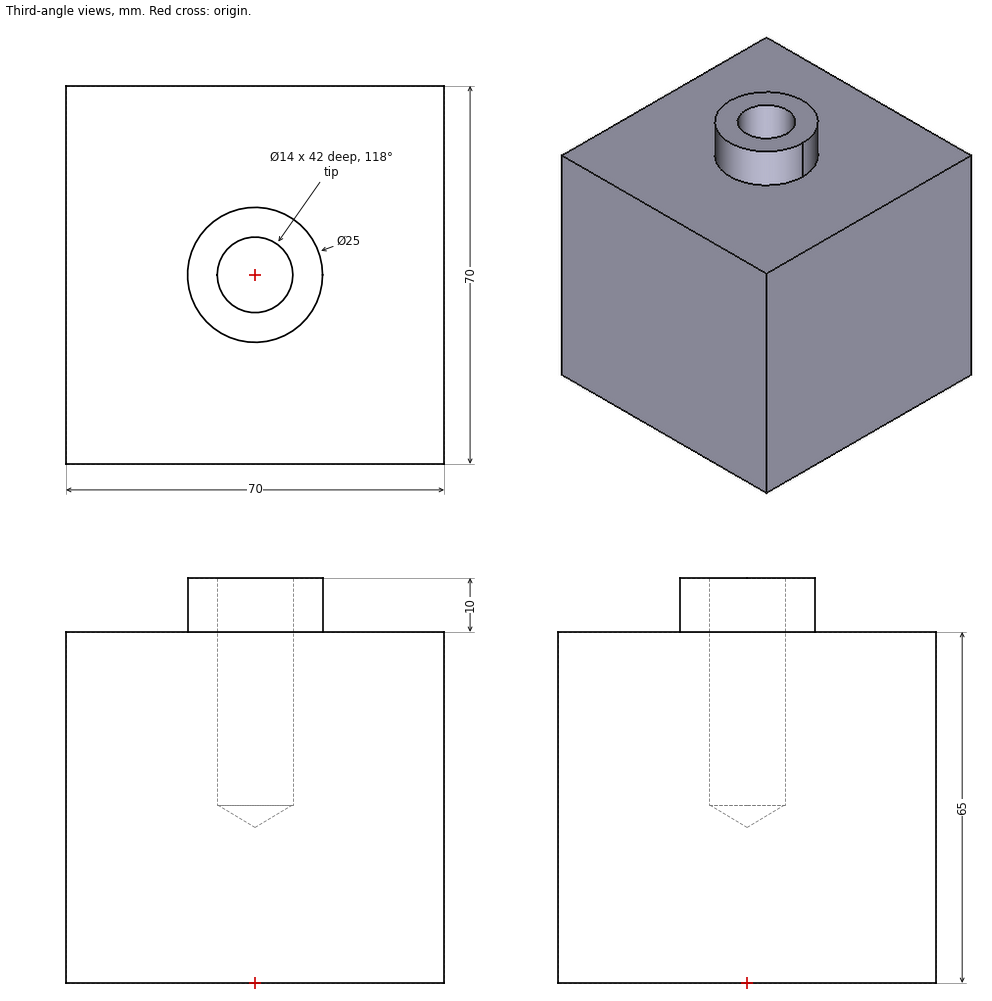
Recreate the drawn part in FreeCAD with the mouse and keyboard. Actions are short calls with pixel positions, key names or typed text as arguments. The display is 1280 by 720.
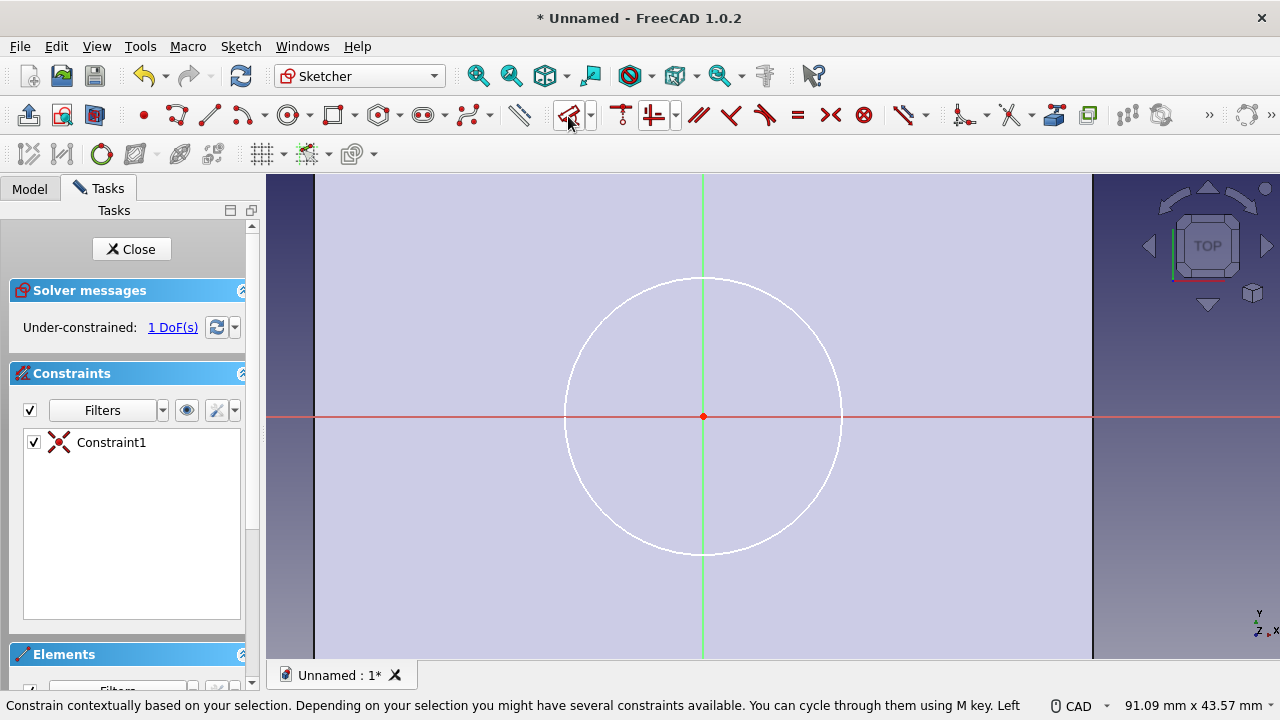
click(801, 318)
click(824, 295)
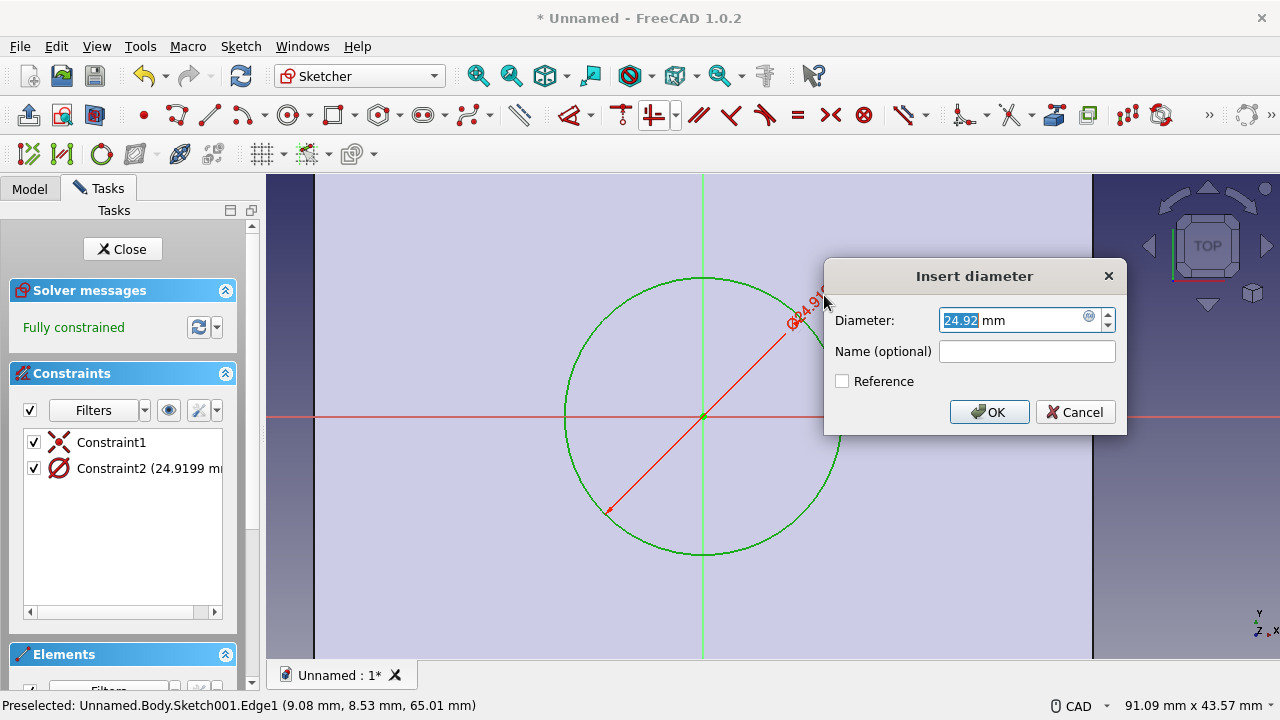
text(25)
key(Return)
key(Escape)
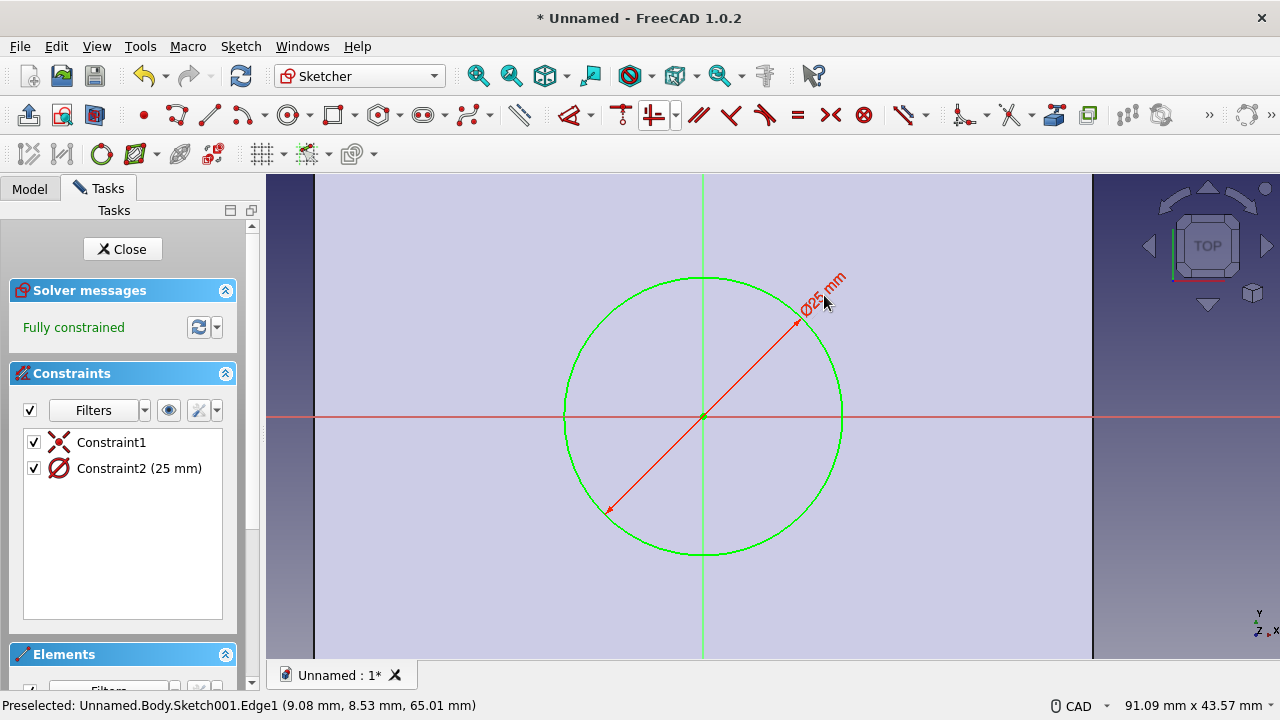
click(123, 249)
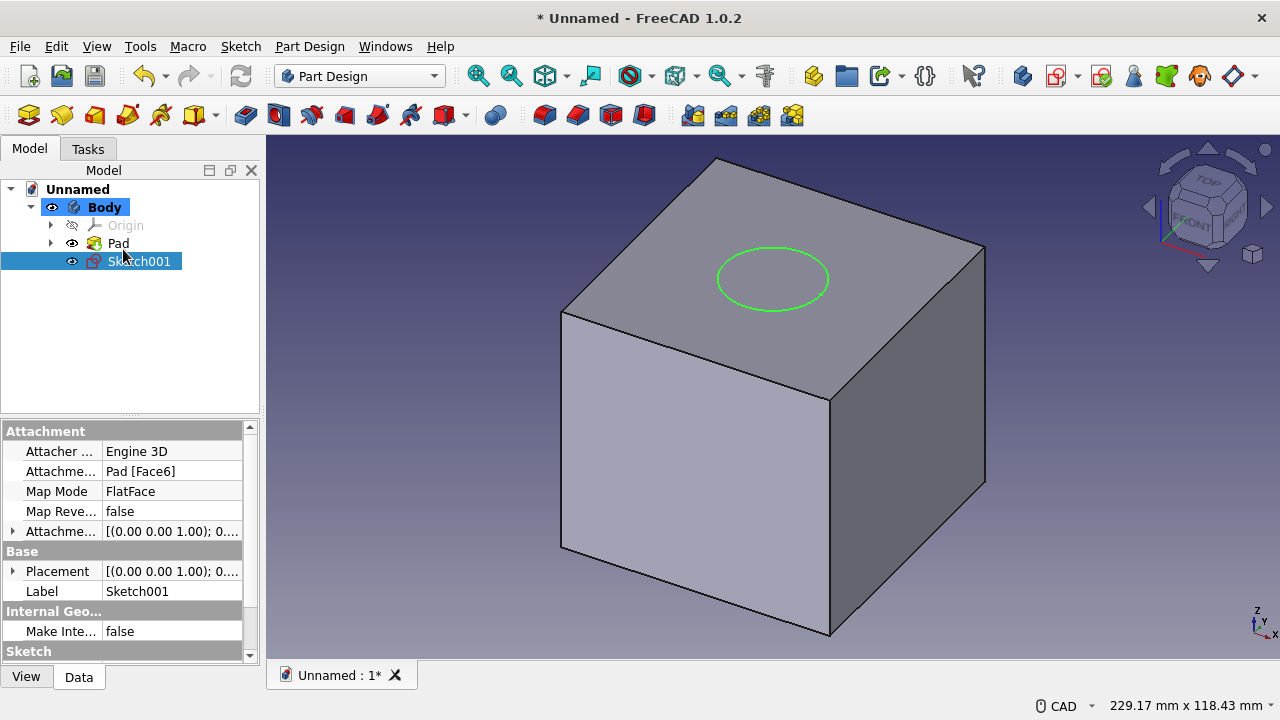
click(29, 116)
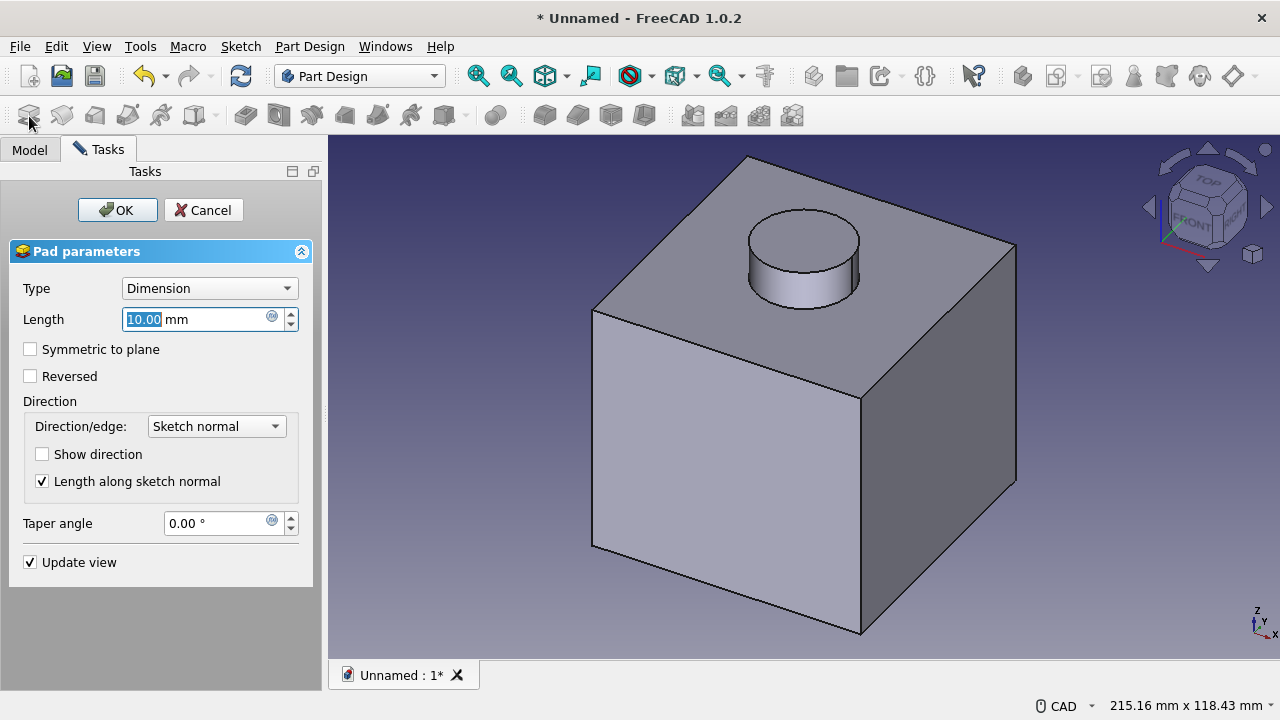
text(10)
key(Tab)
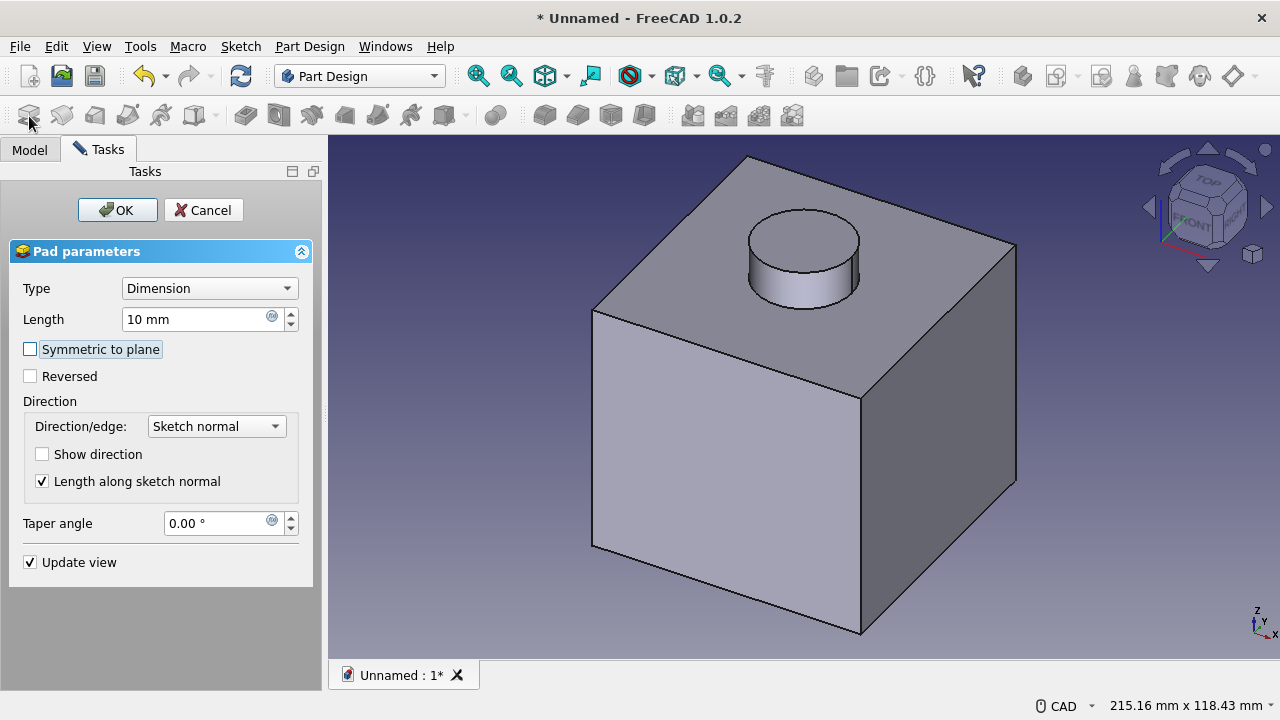
click(118, 210)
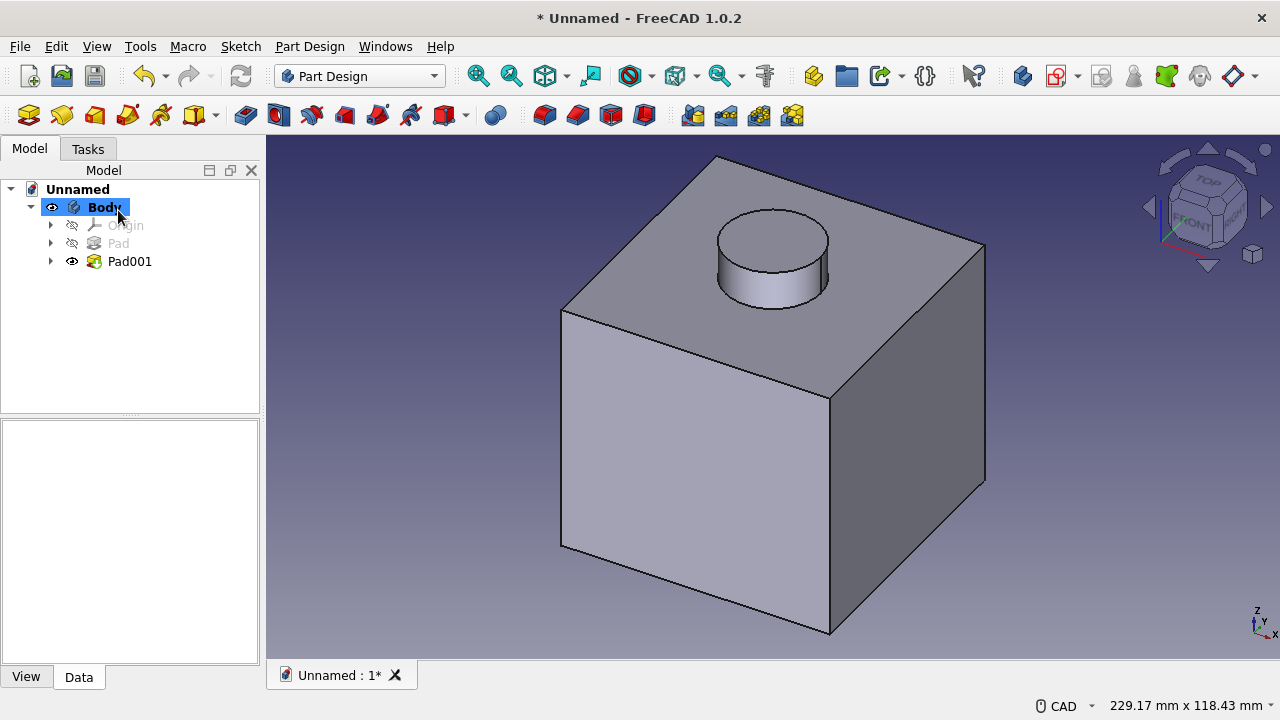
click(479, 76)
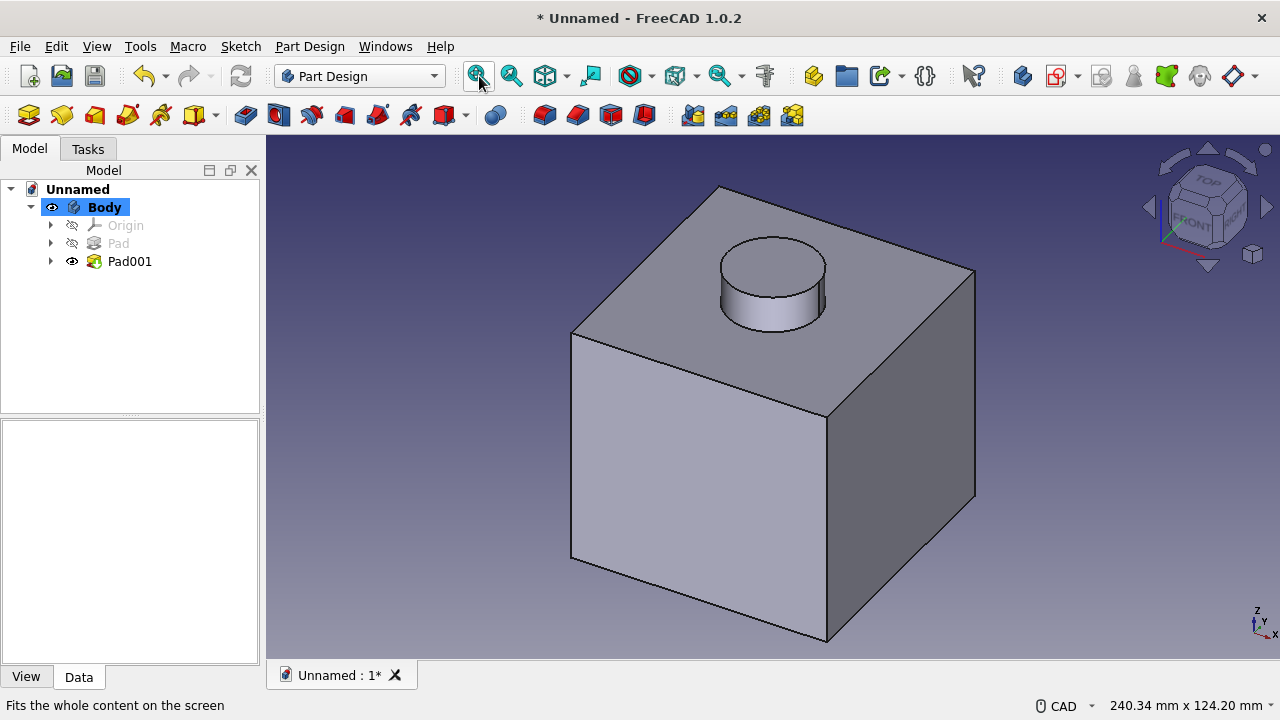
click(773, 266)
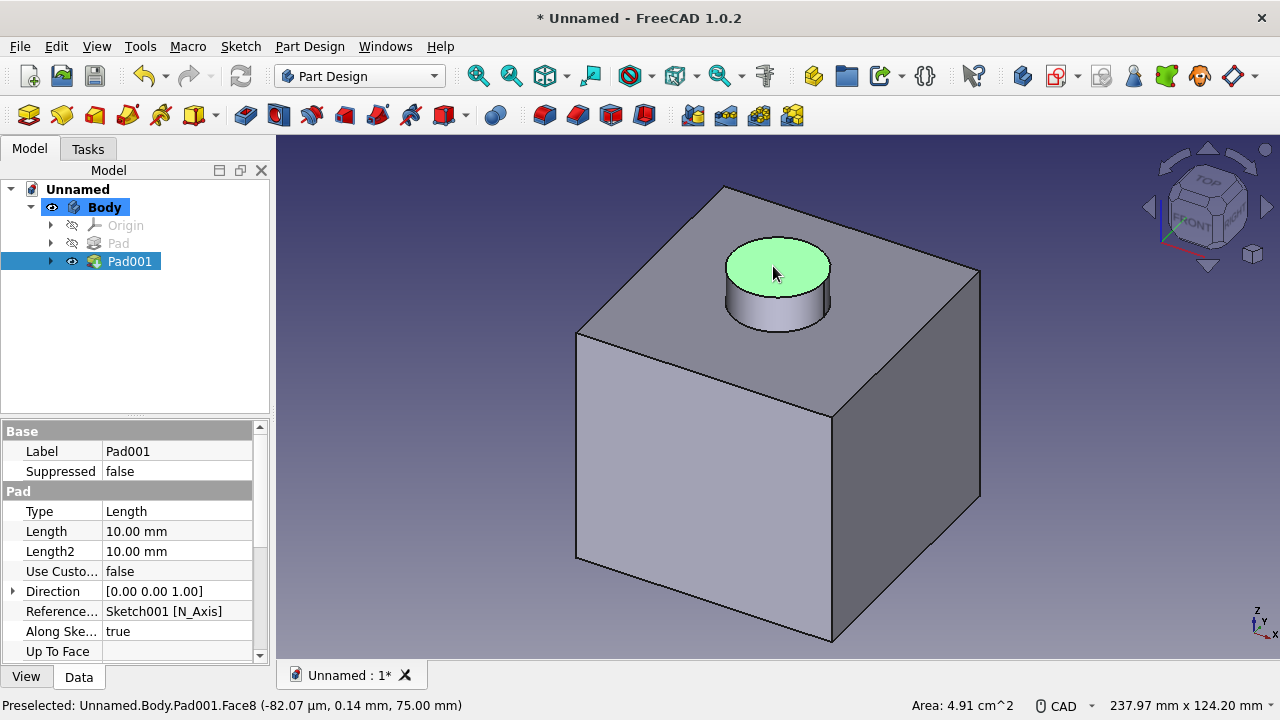
click(1056, 76)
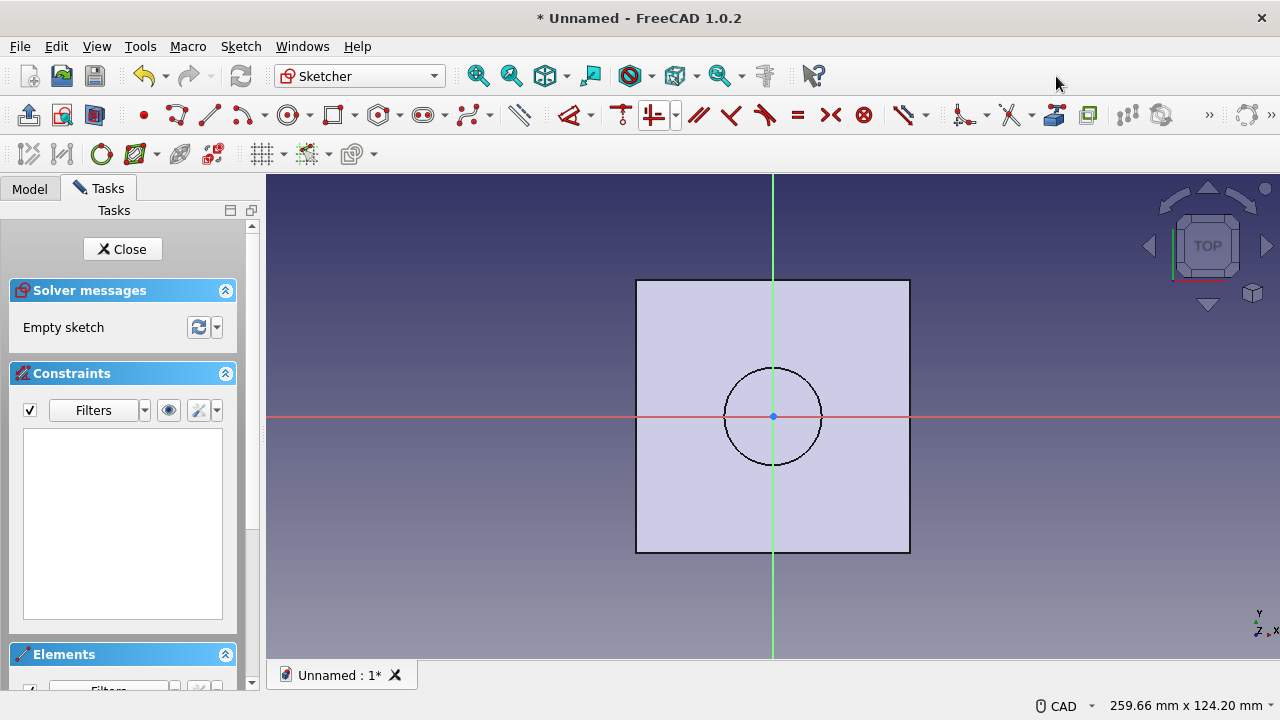
scroll(787, 416, up, 9)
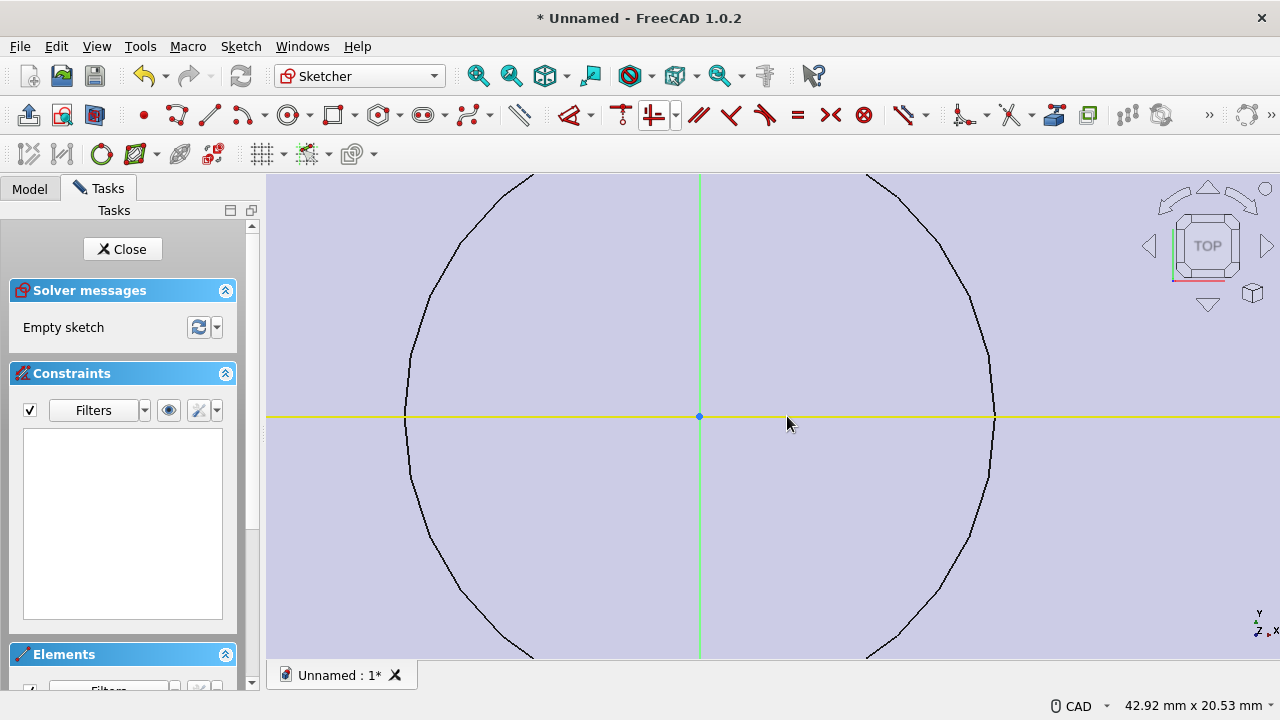
click(288, 116)